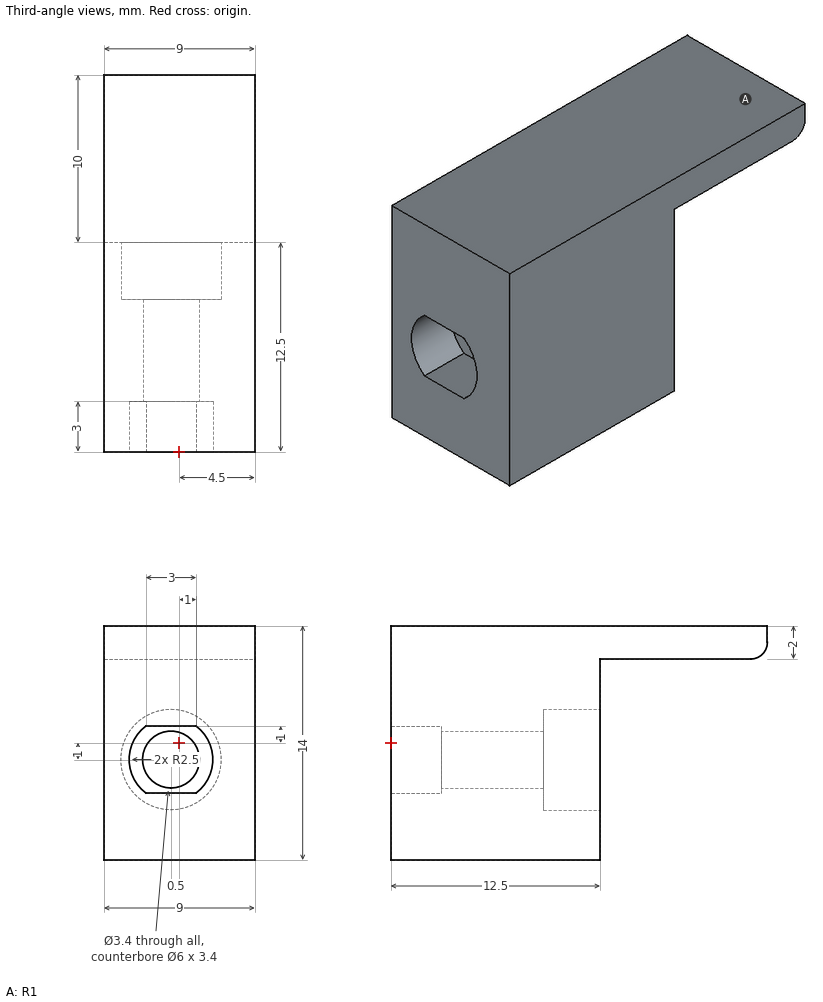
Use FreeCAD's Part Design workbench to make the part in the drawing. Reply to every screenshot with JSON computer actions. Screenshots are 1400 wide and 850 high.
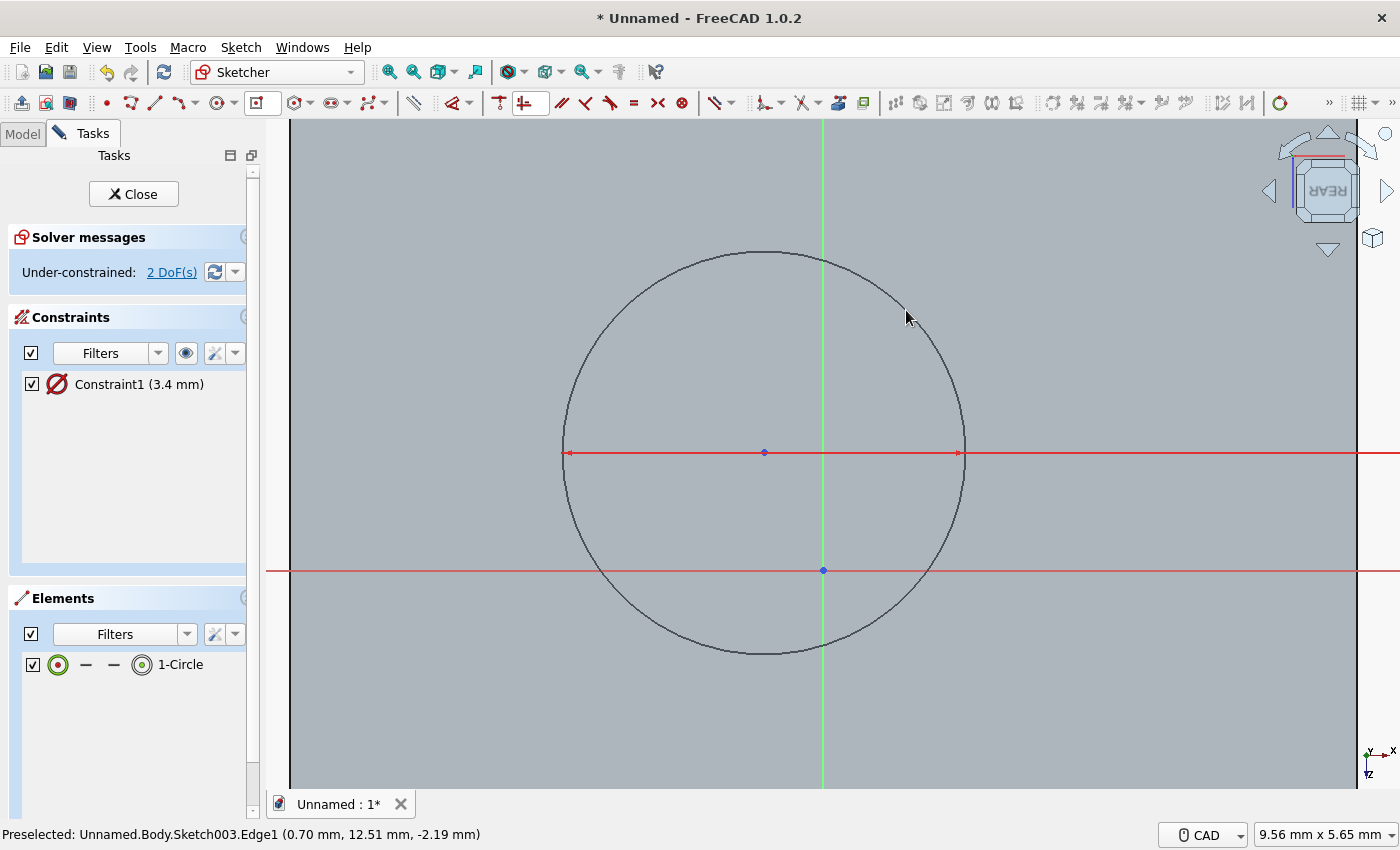
{"action": "key", "text": "d"}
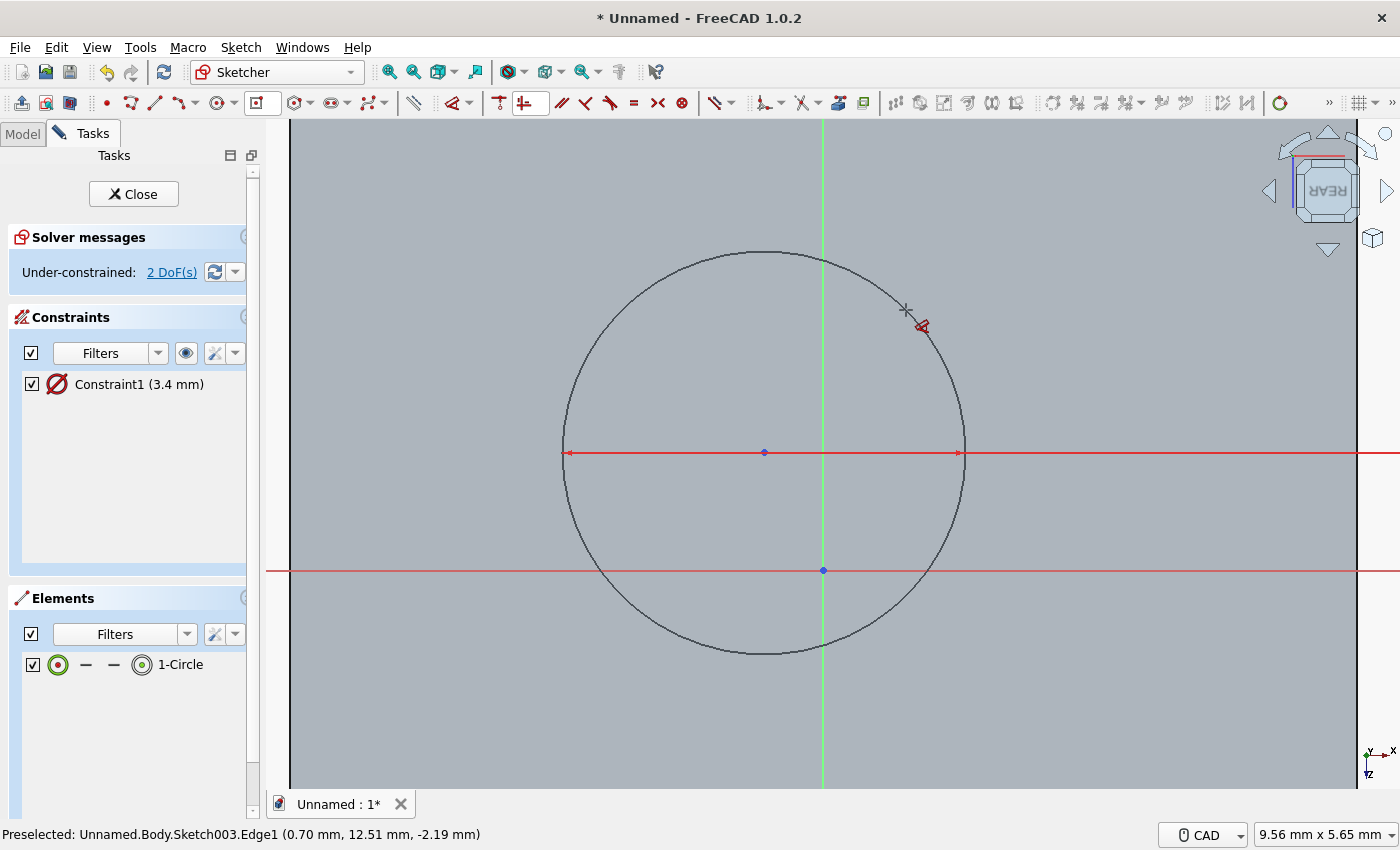
{"action": "left_click", "coordinate": [764, 453]}
{"action": "left_click", "coordinate": [857, 512]}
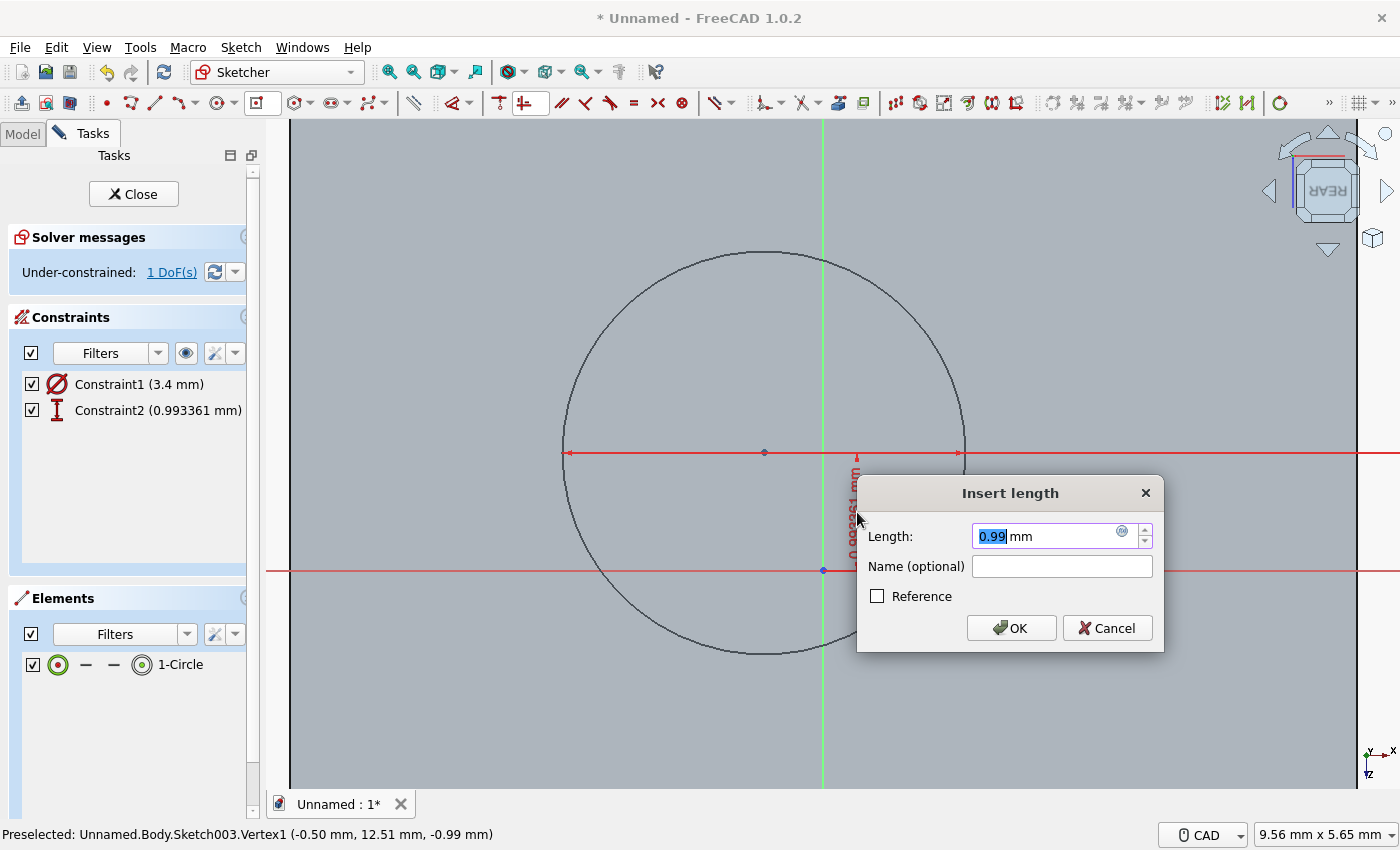
{"action": "type", "text": "1"}
{"action": "key", "text": "Return"}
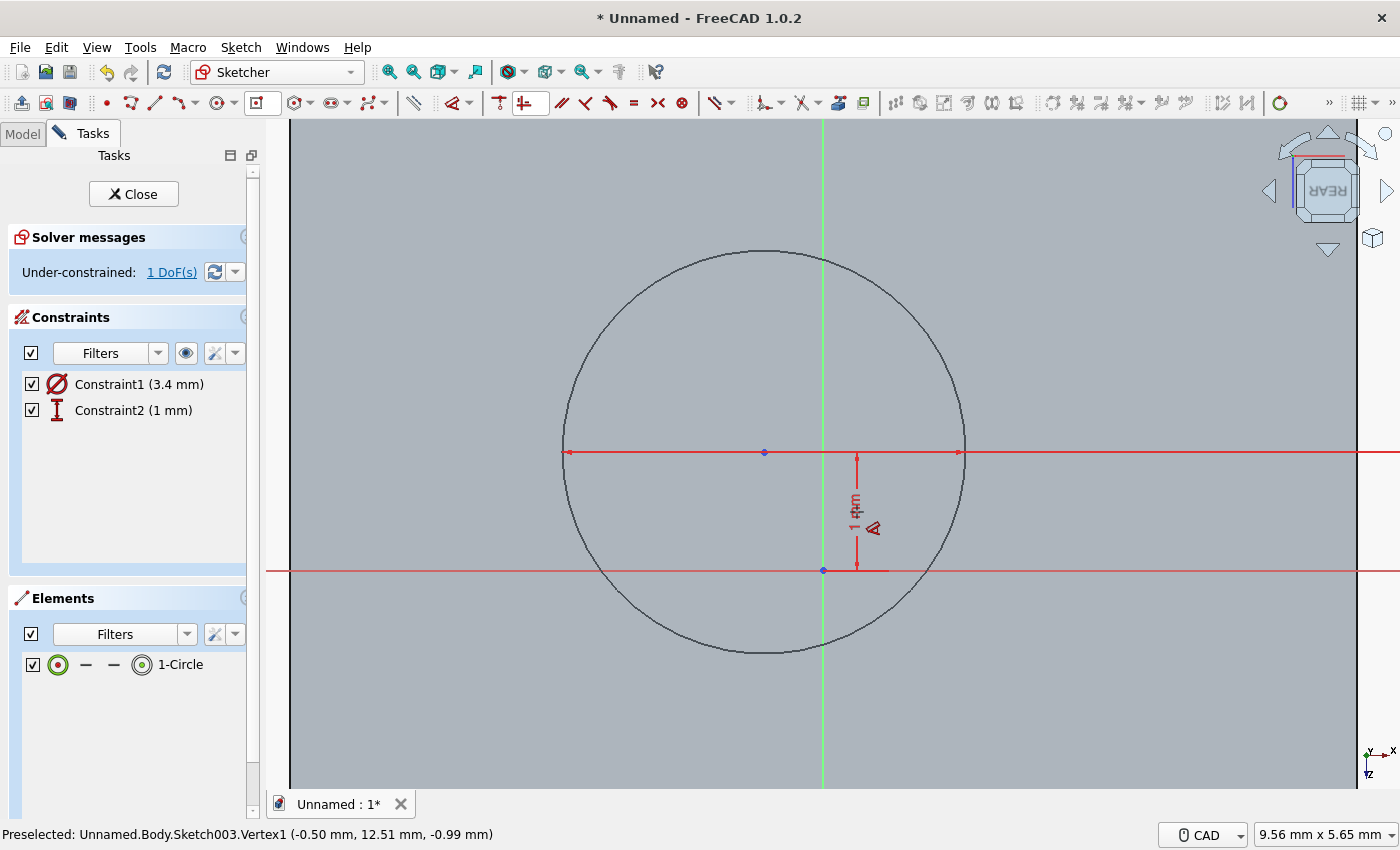
{"action": "left_click", "coordinate": [764, 452]}
{"action": "left_click", "coordinate": [794, 605]}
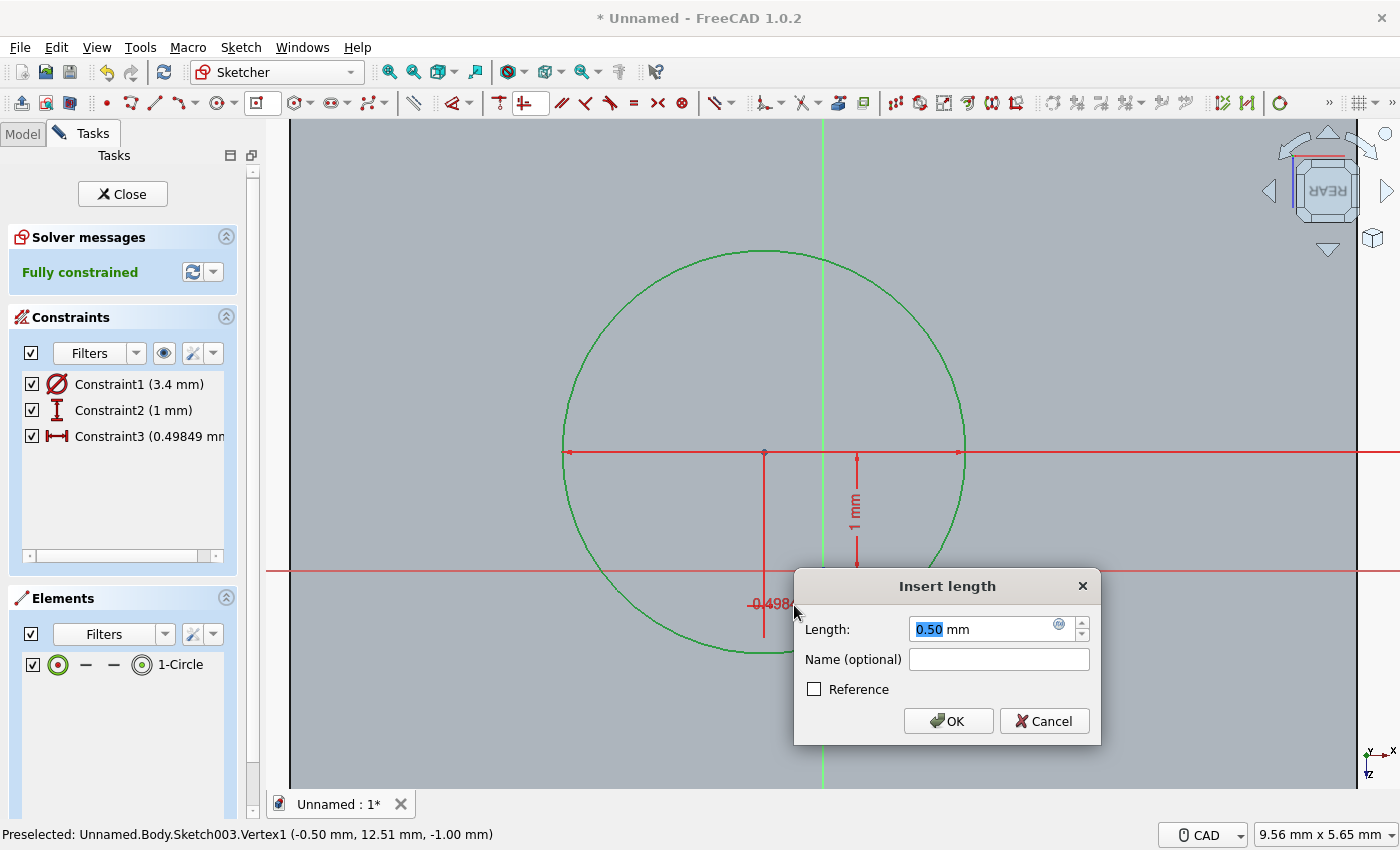
{"action": "type", "text": "0.5"}
{"action": "key", "text": "Return"}
{"action": "key", "text": "Escape"}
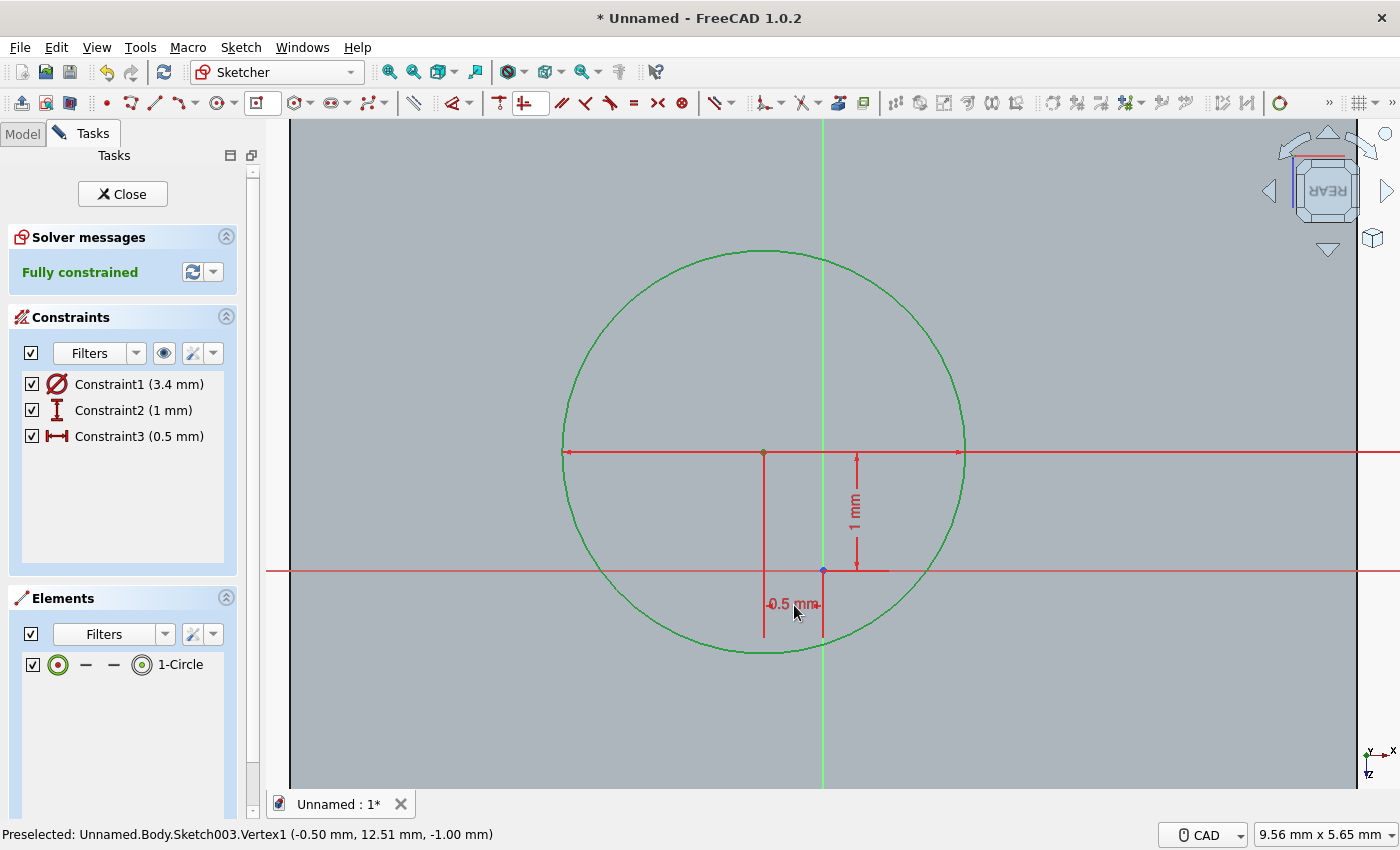
{"action": "left_click", "coordinate": [123, 194]}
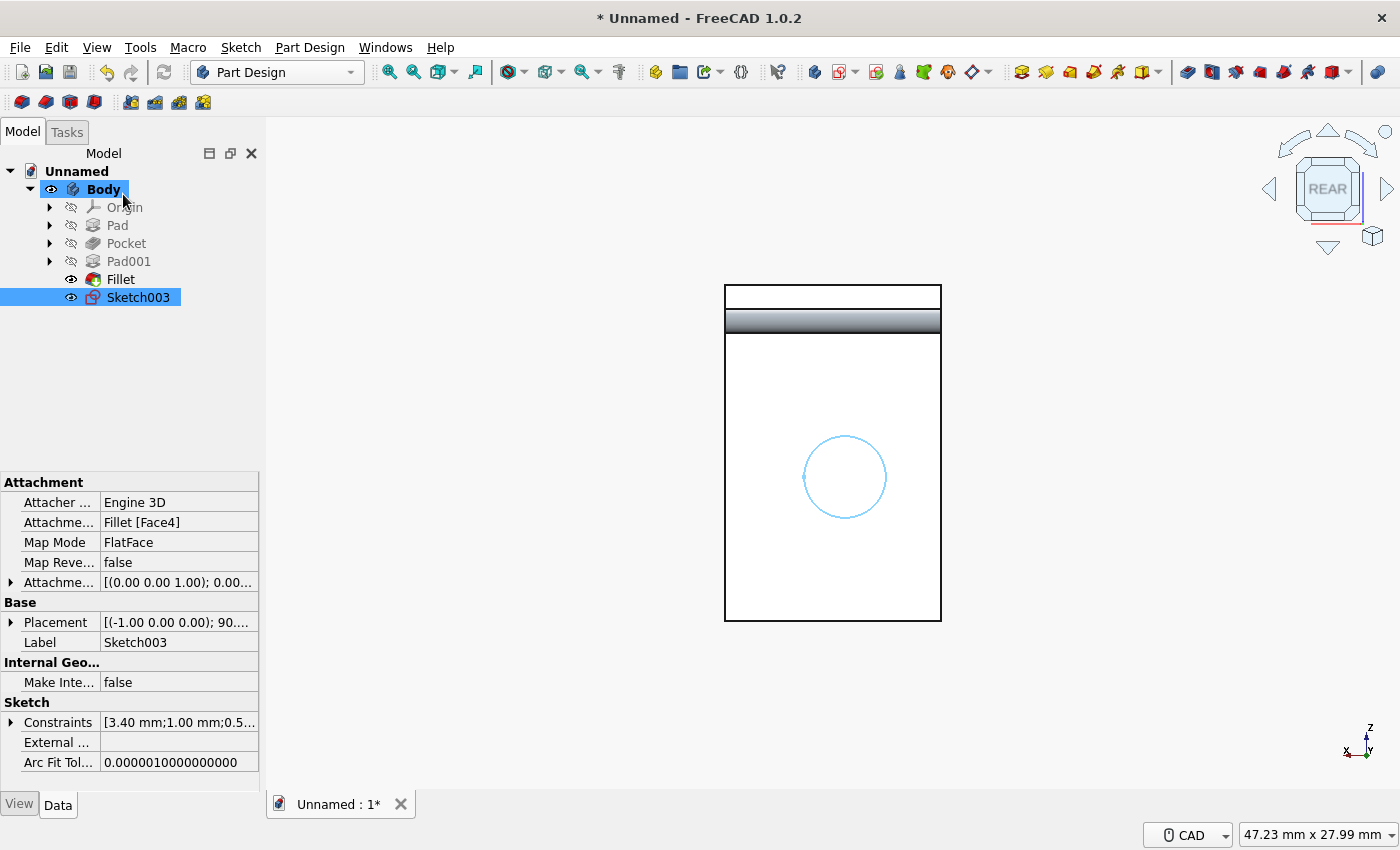
{"action": "left_click", "coordinate": [1212, 72]}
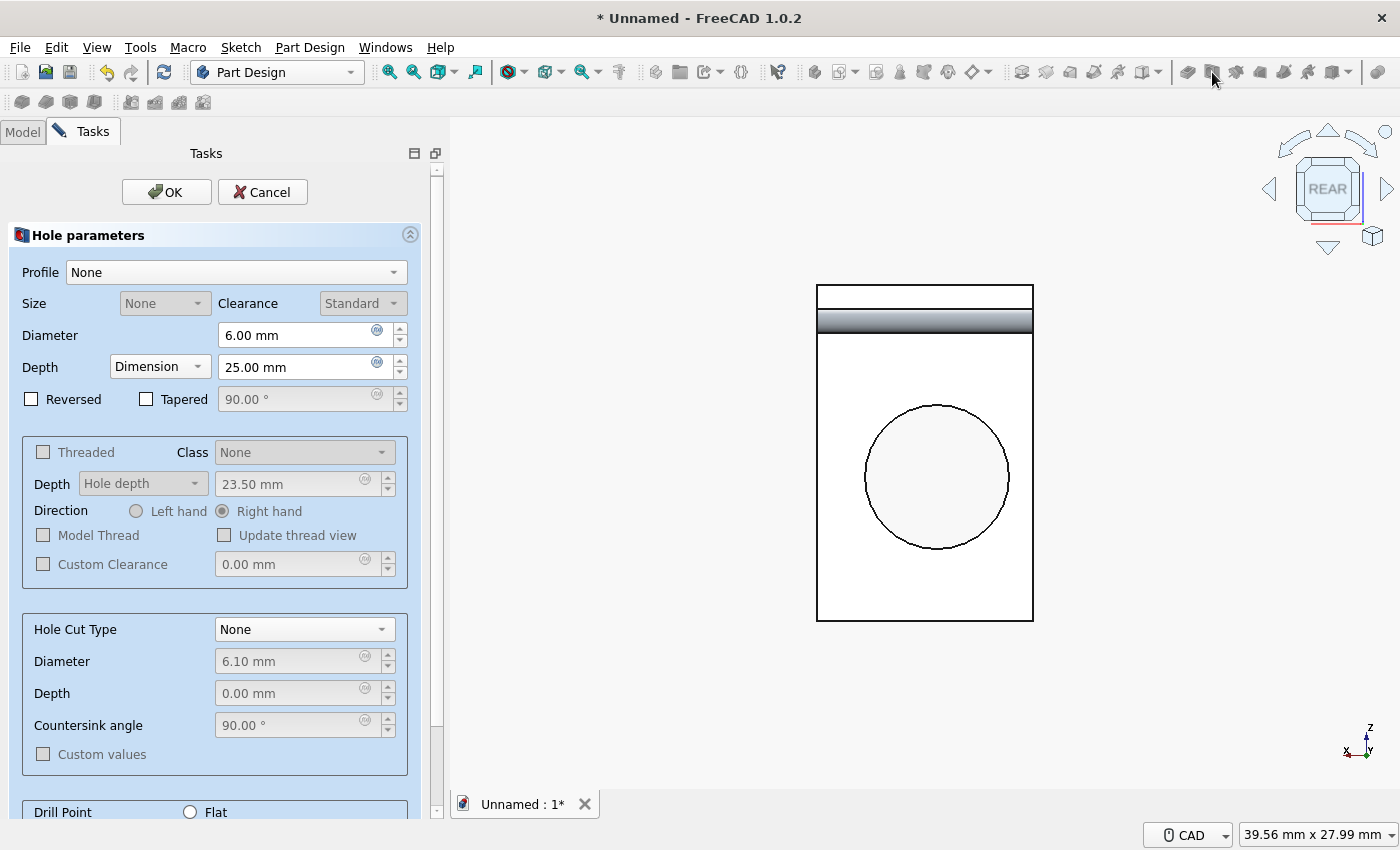
{"action": "triple_click", "coordinate": [305, 335]}